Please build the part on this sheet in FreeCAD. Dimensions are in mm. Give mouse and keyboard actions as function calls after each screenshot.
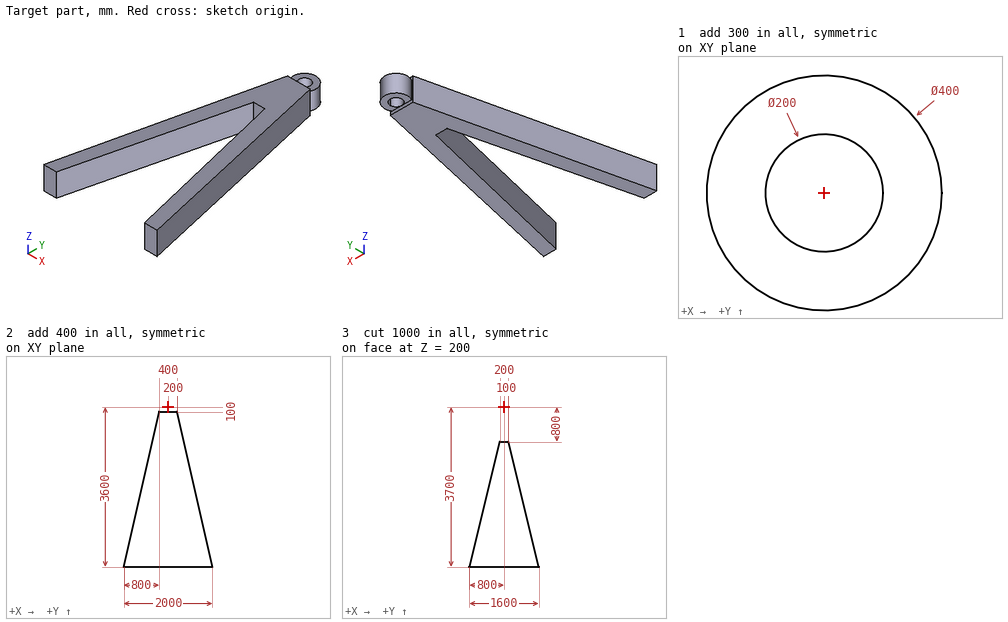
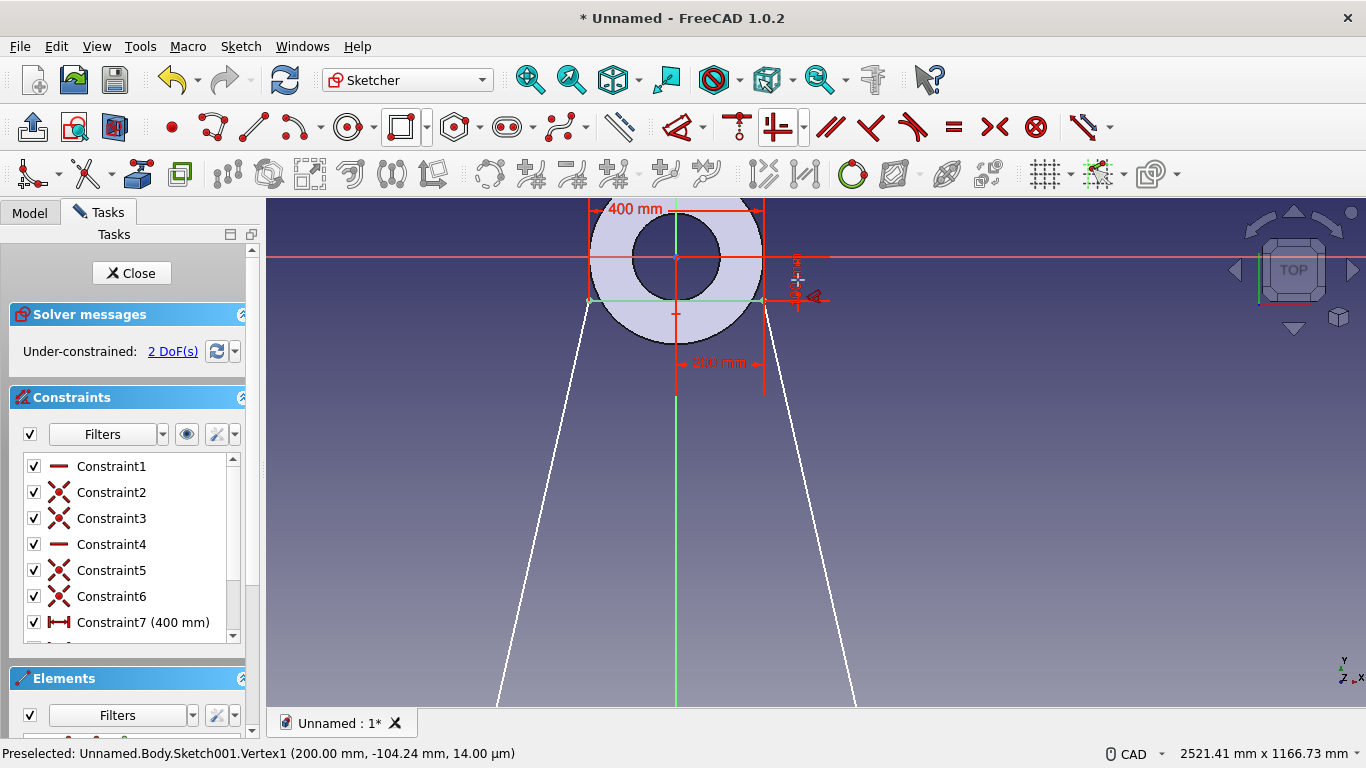
scroll(766, 303, down, 8)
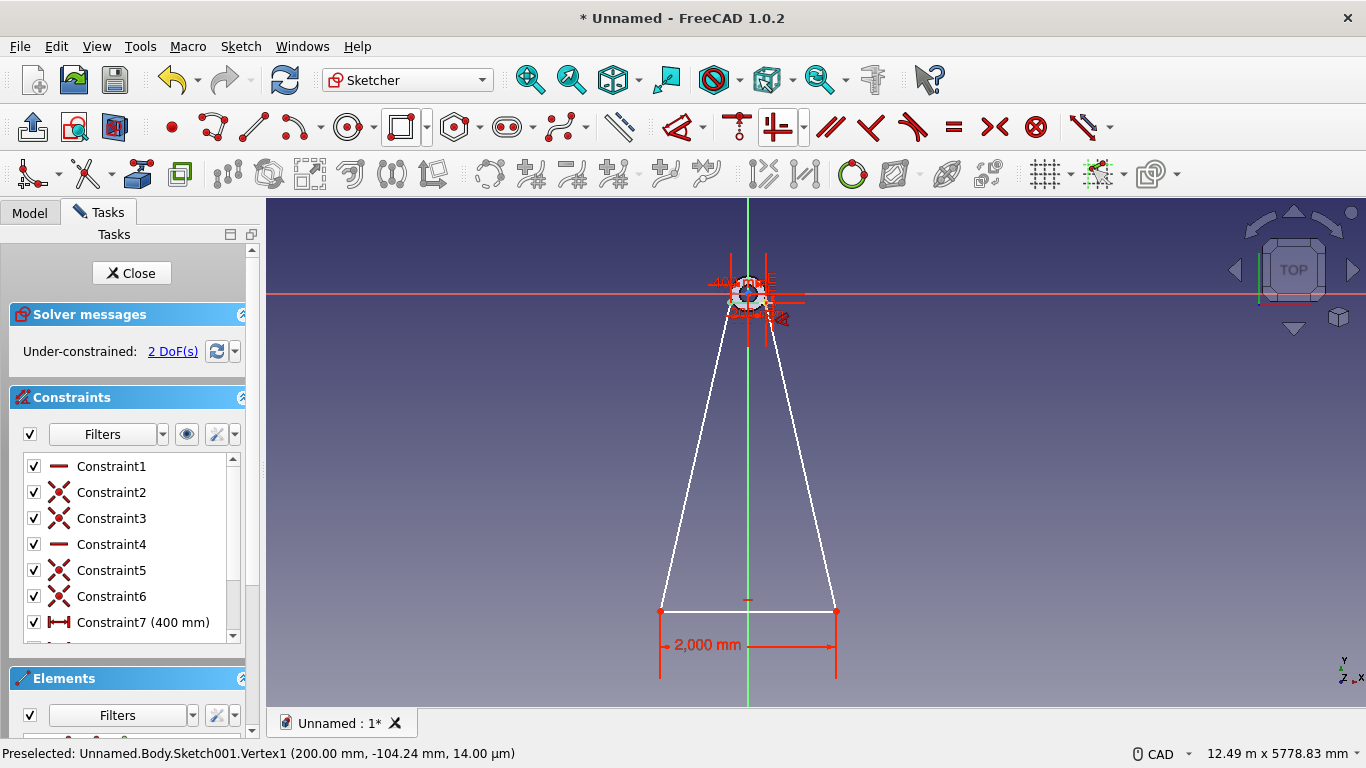
click(717, 365)
click(695, 670)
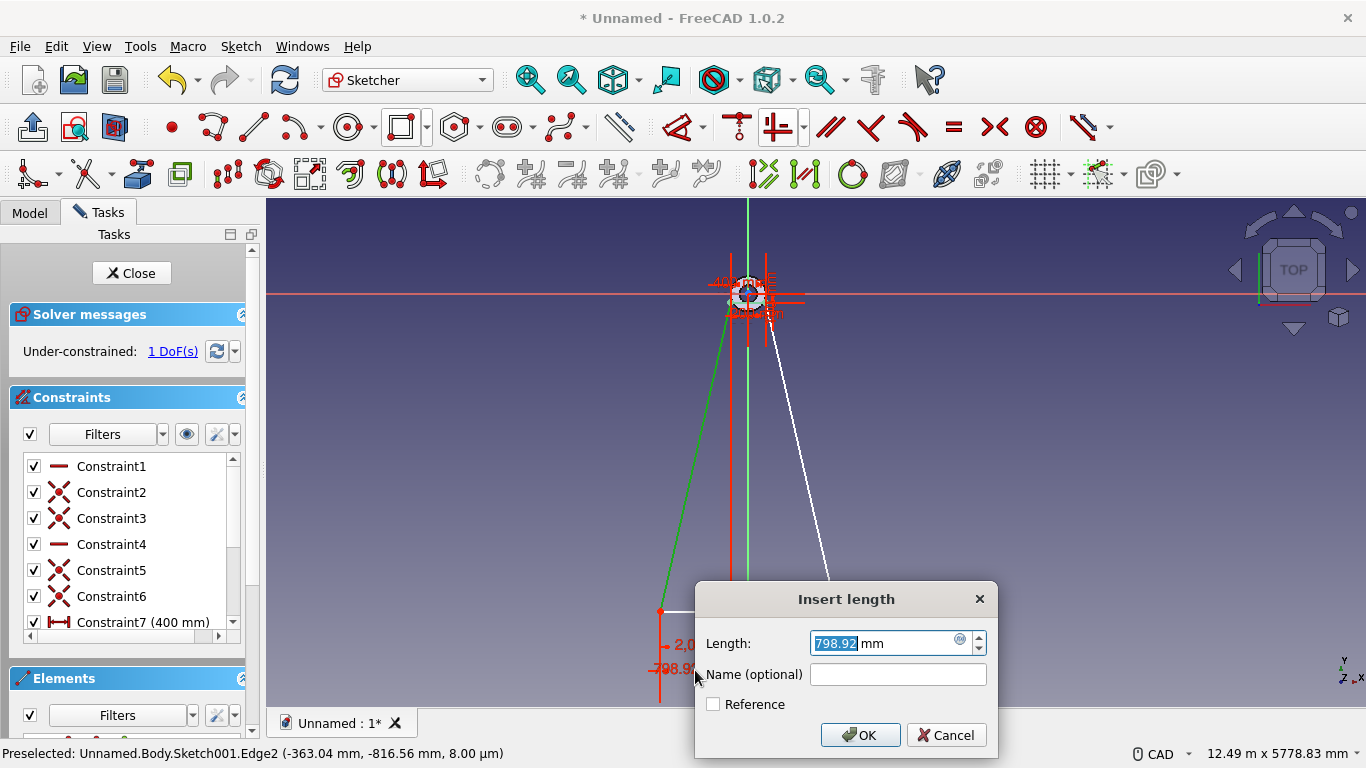
text(800)
key(Return)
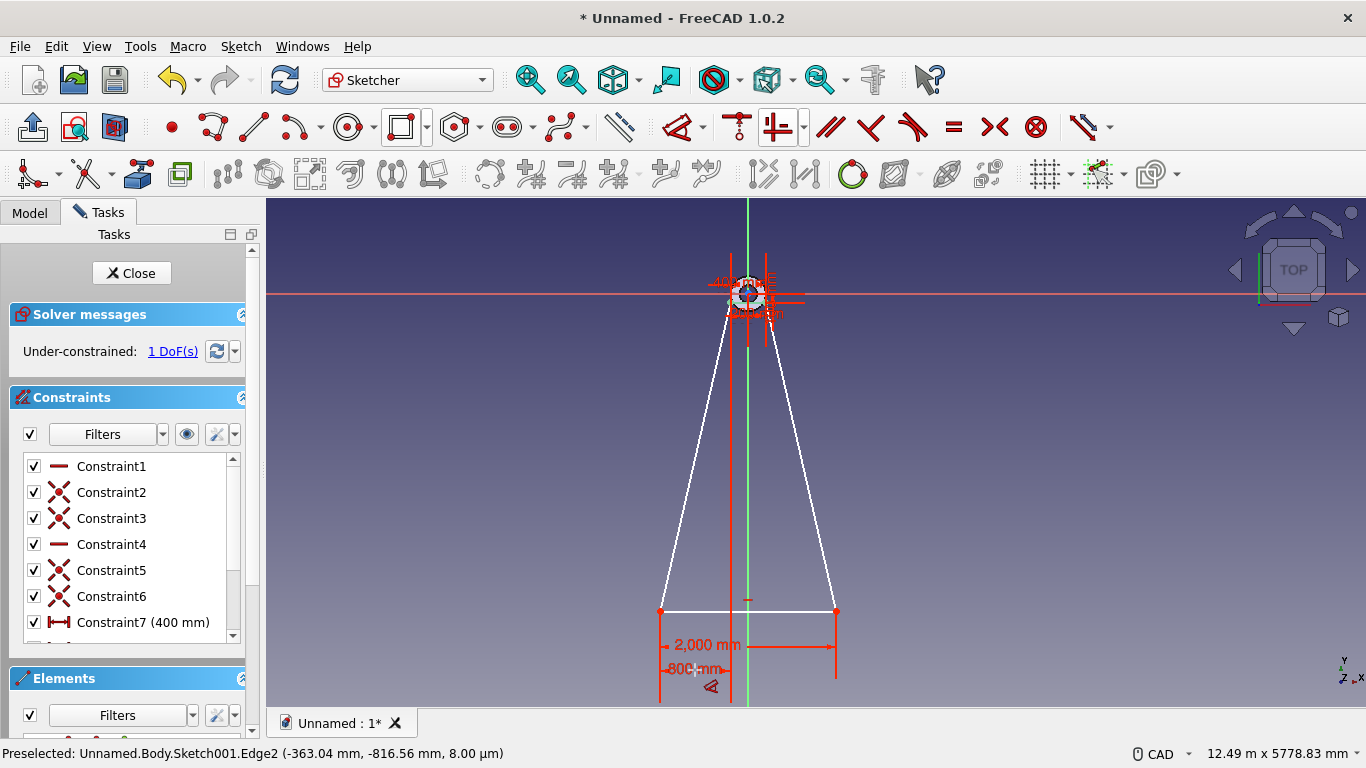
click(660, 612)
click(626, 453)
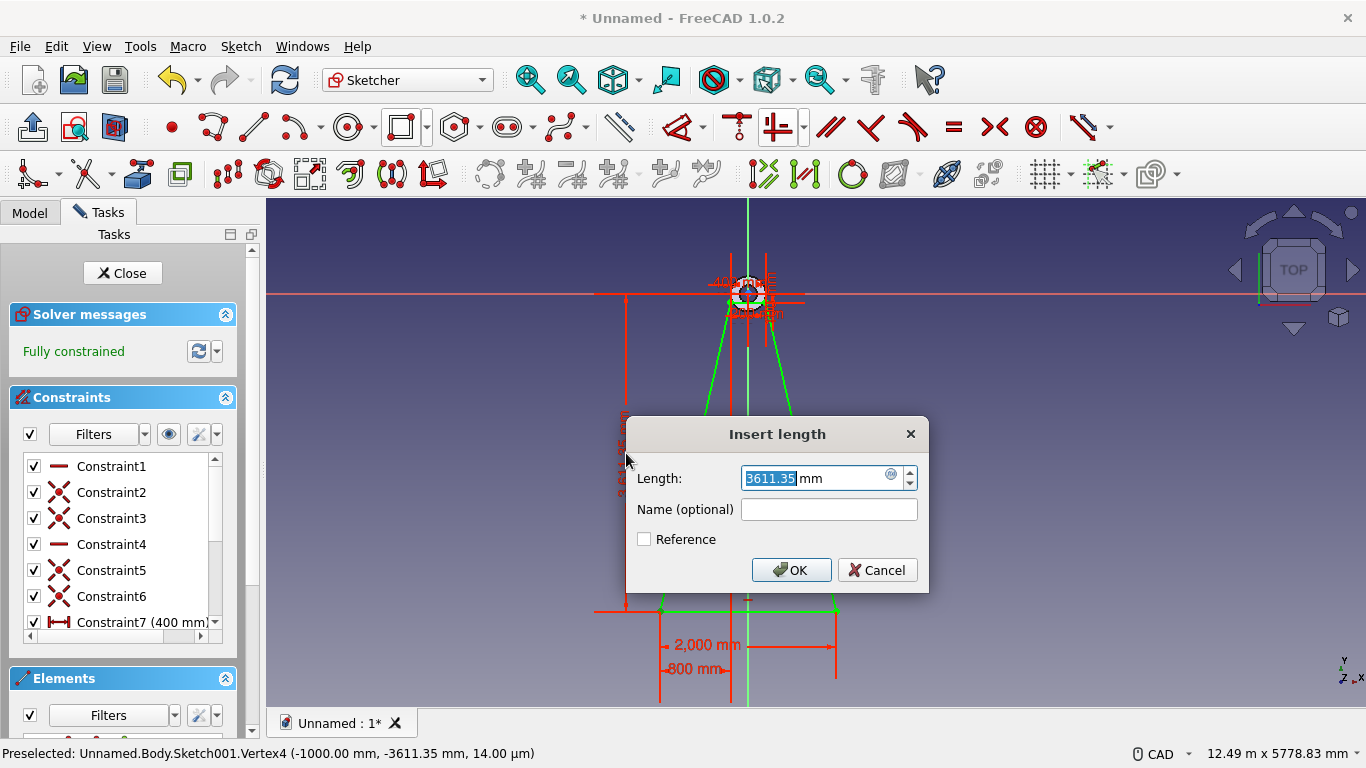
text(3600)
key(Return)
key(Escape)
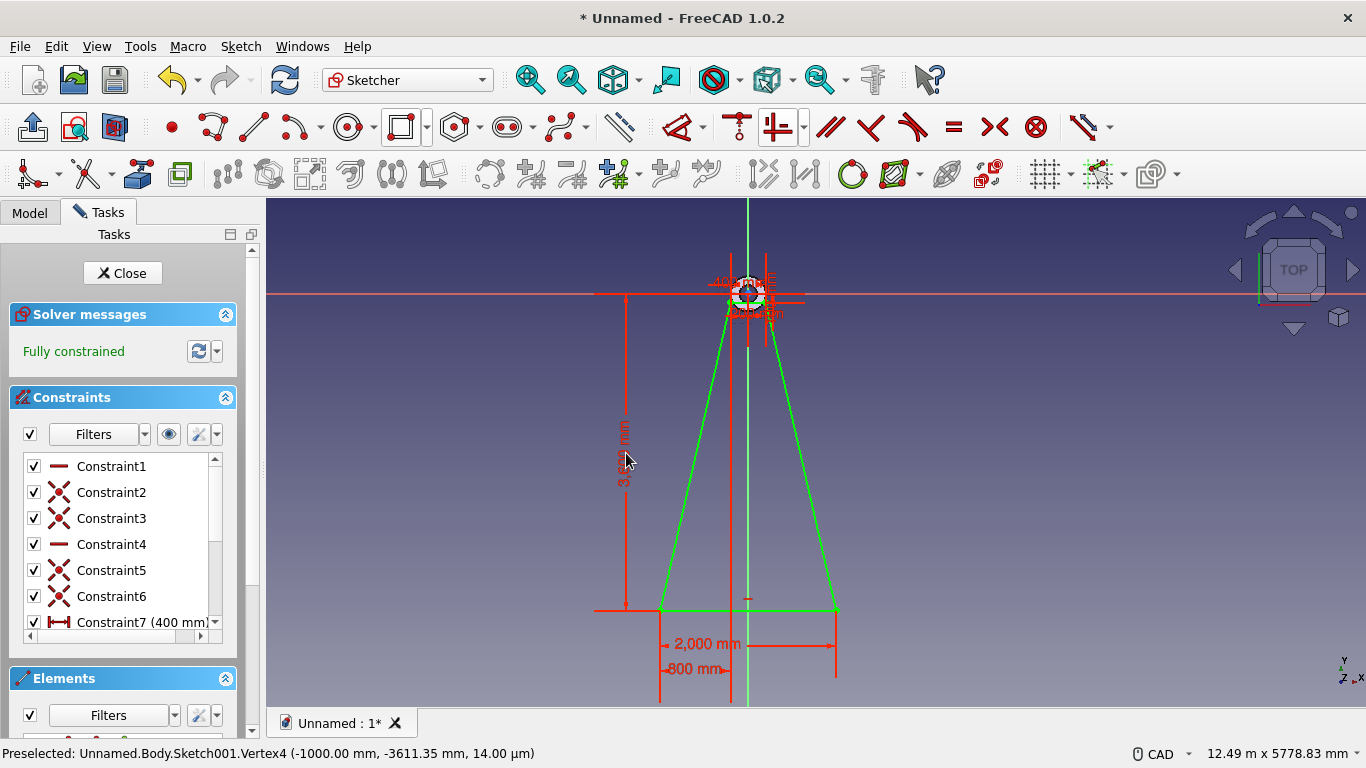
click(123, 273)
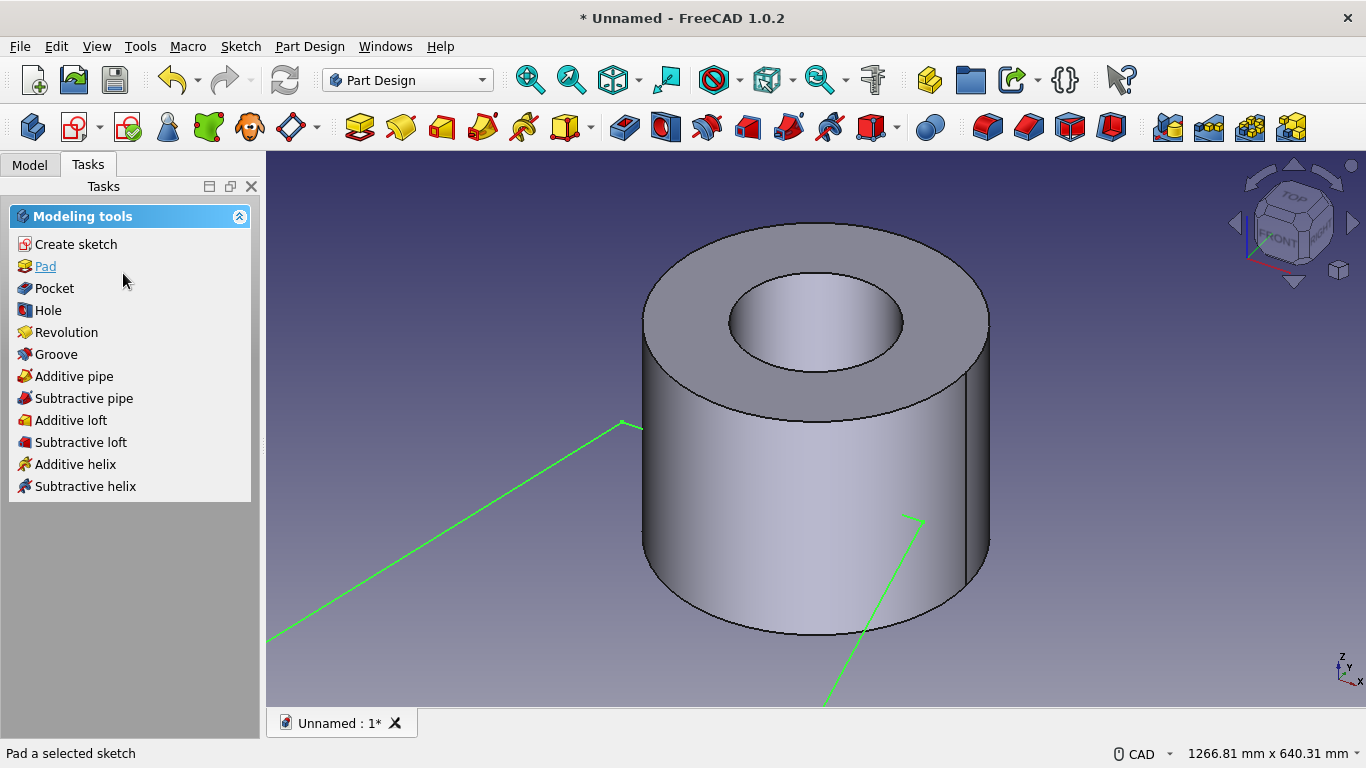
click(360, 128)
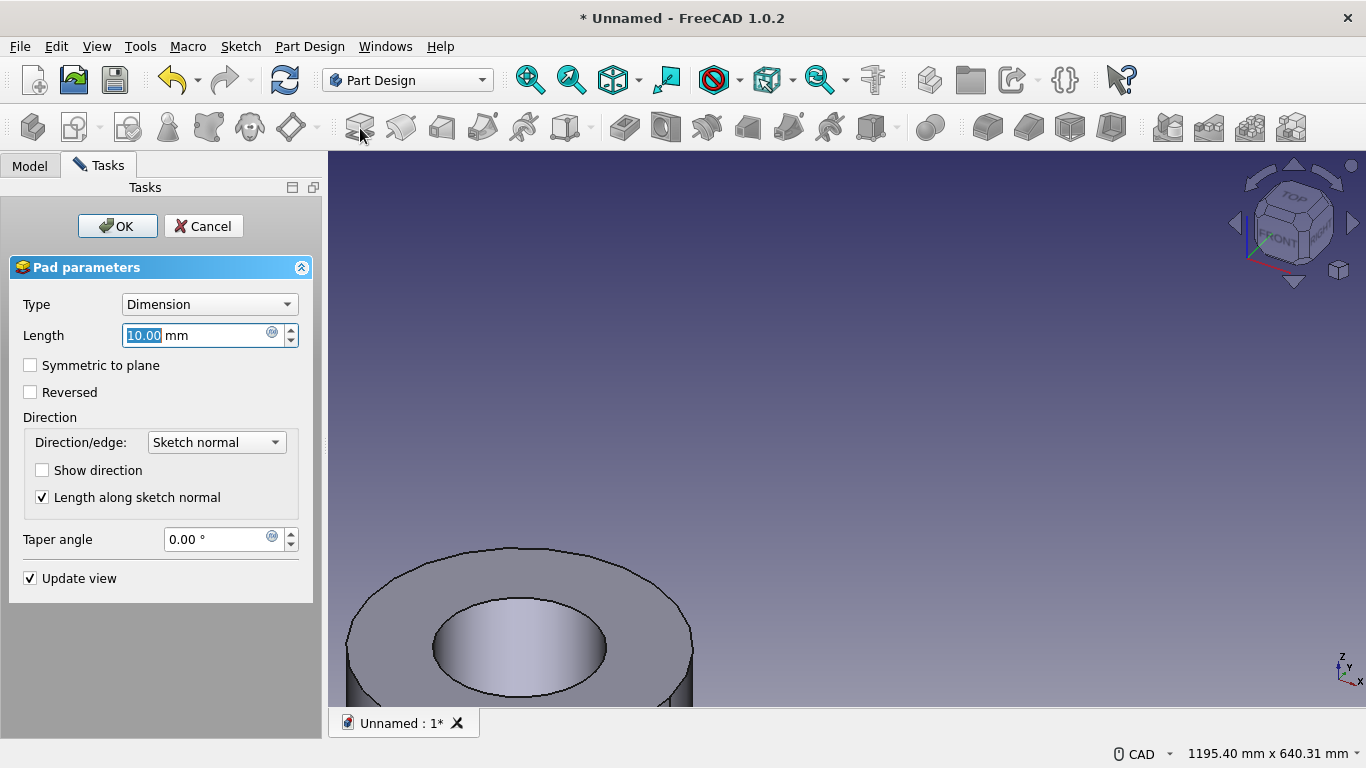
text(400)
key(Tab)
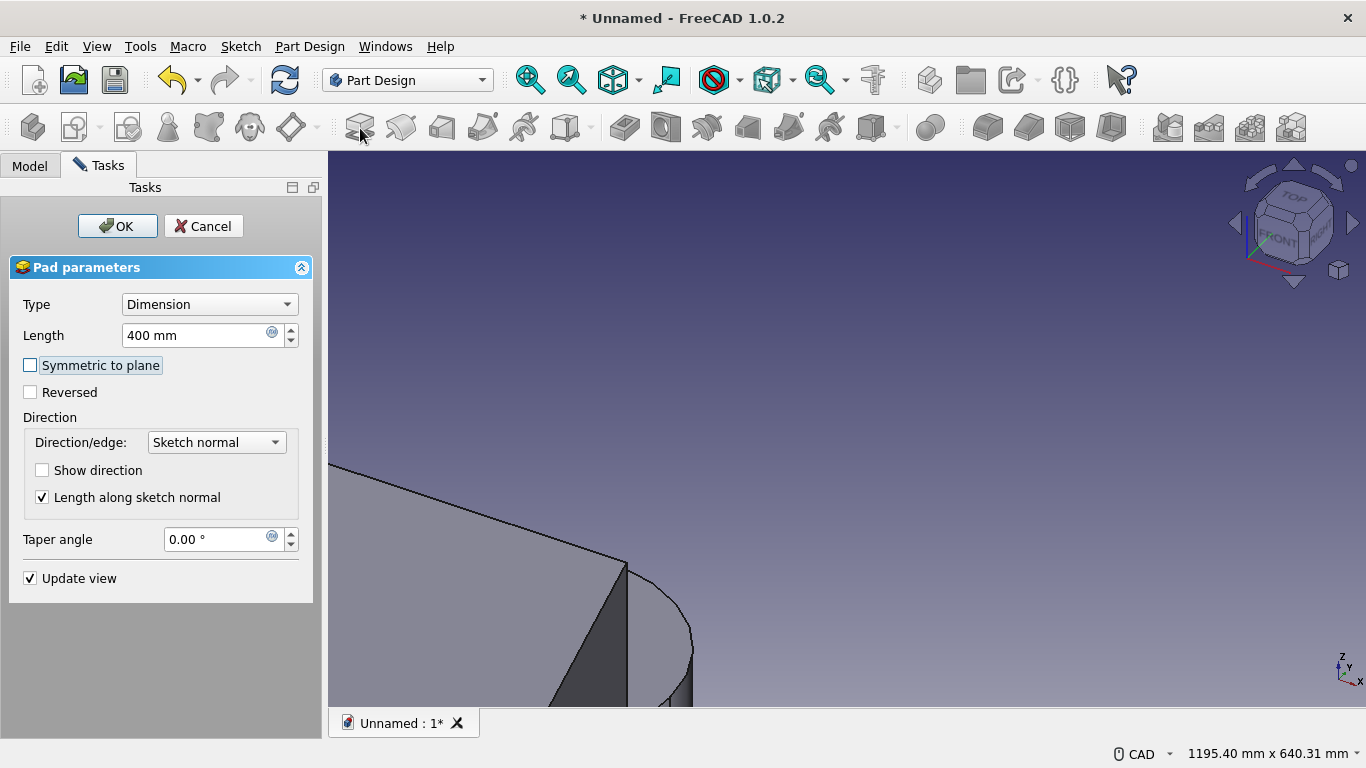
click(31, 365)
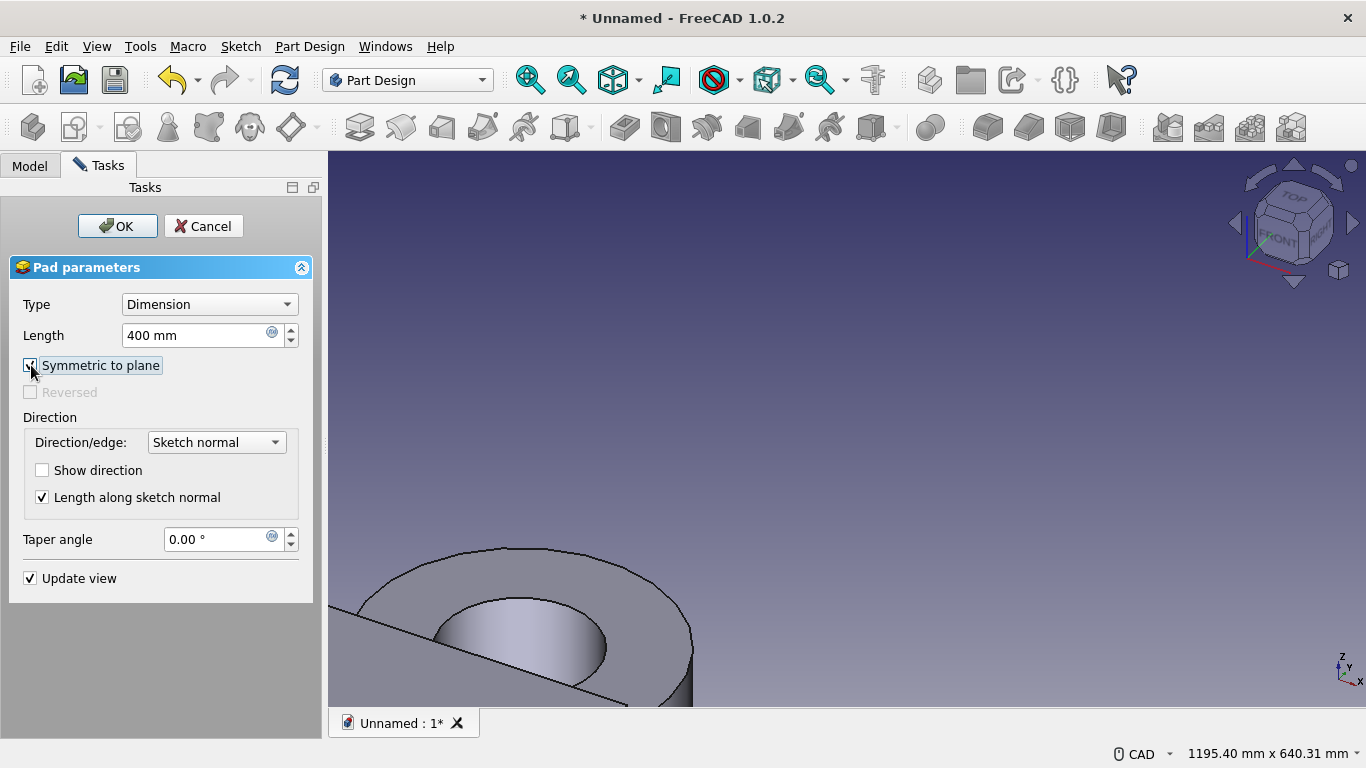
click(118, 226)